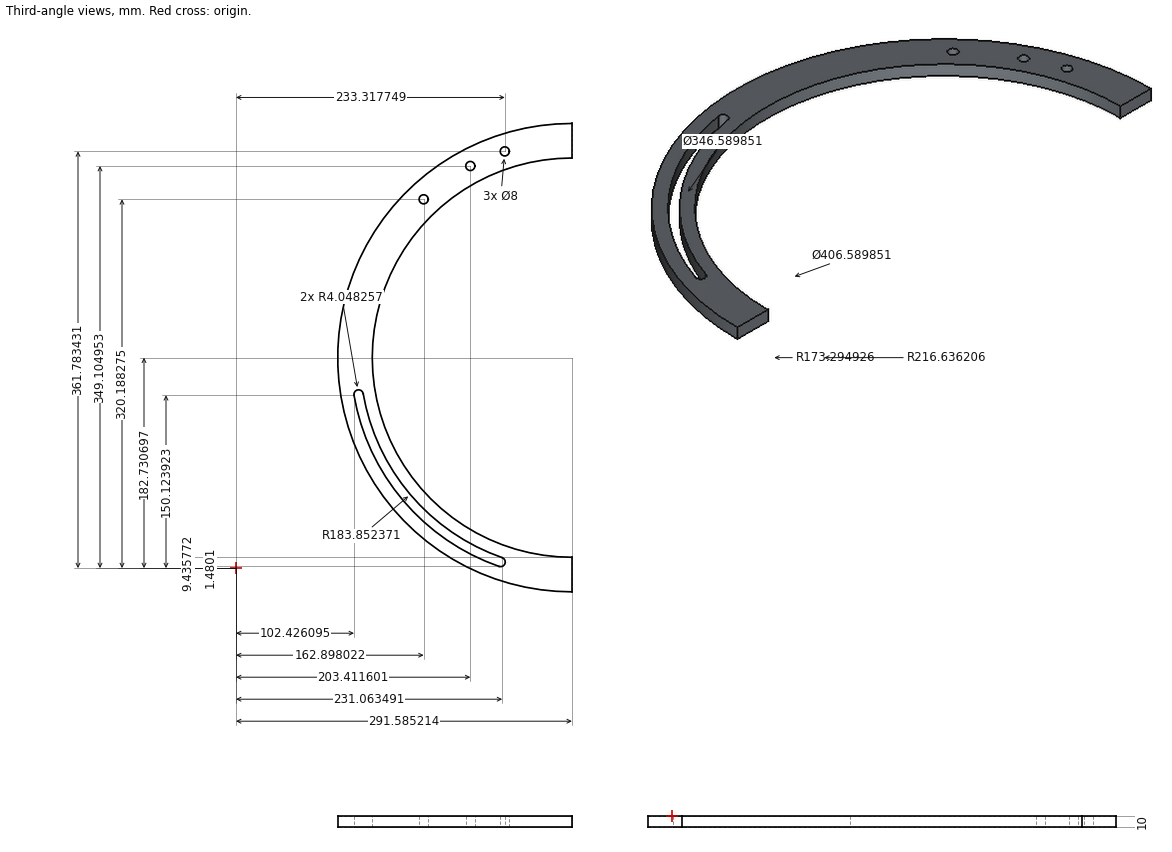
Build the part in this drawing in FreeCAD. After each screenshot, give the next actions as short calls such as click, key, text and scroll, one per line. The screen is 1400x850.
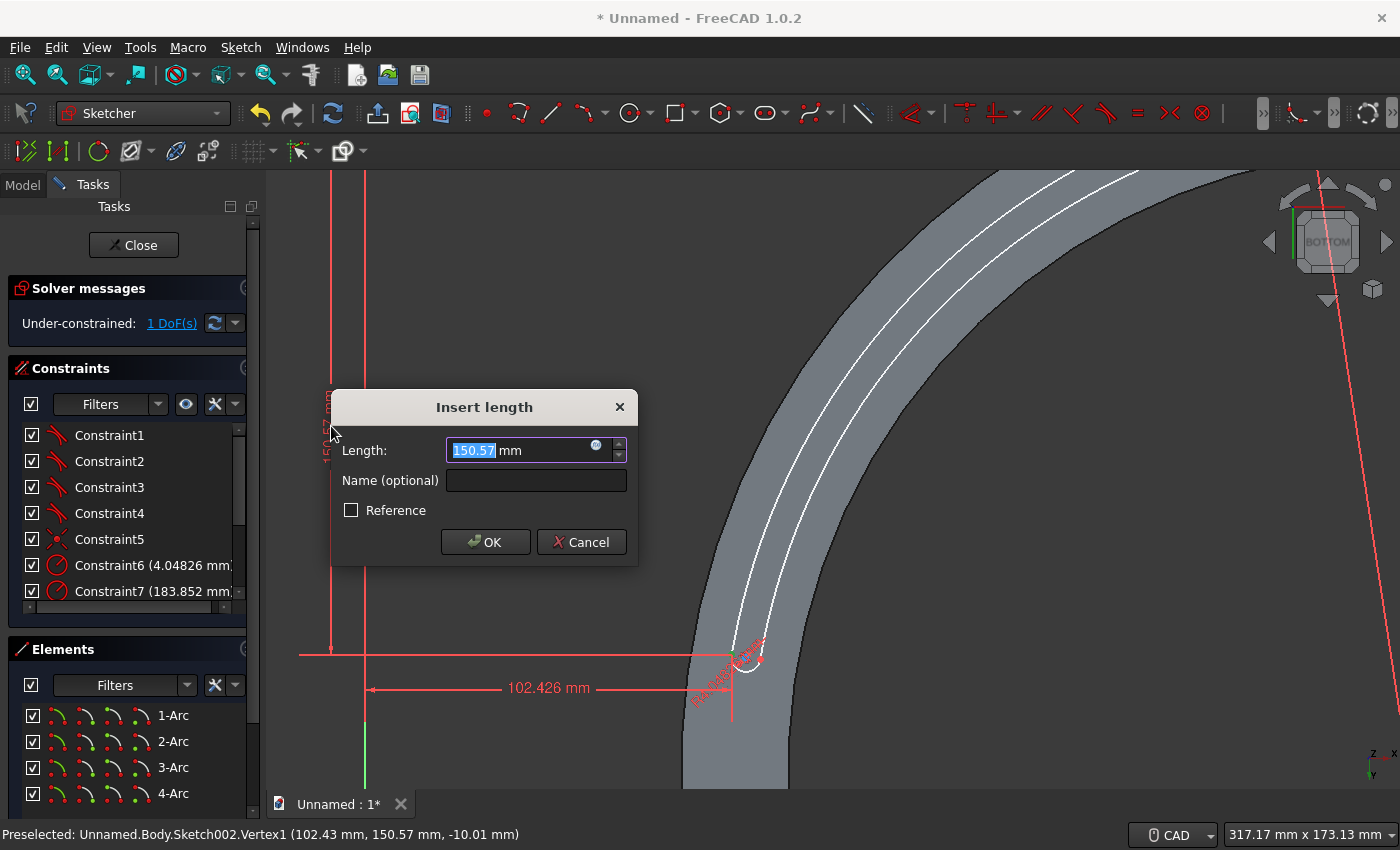
text(150.123923)
key(Return)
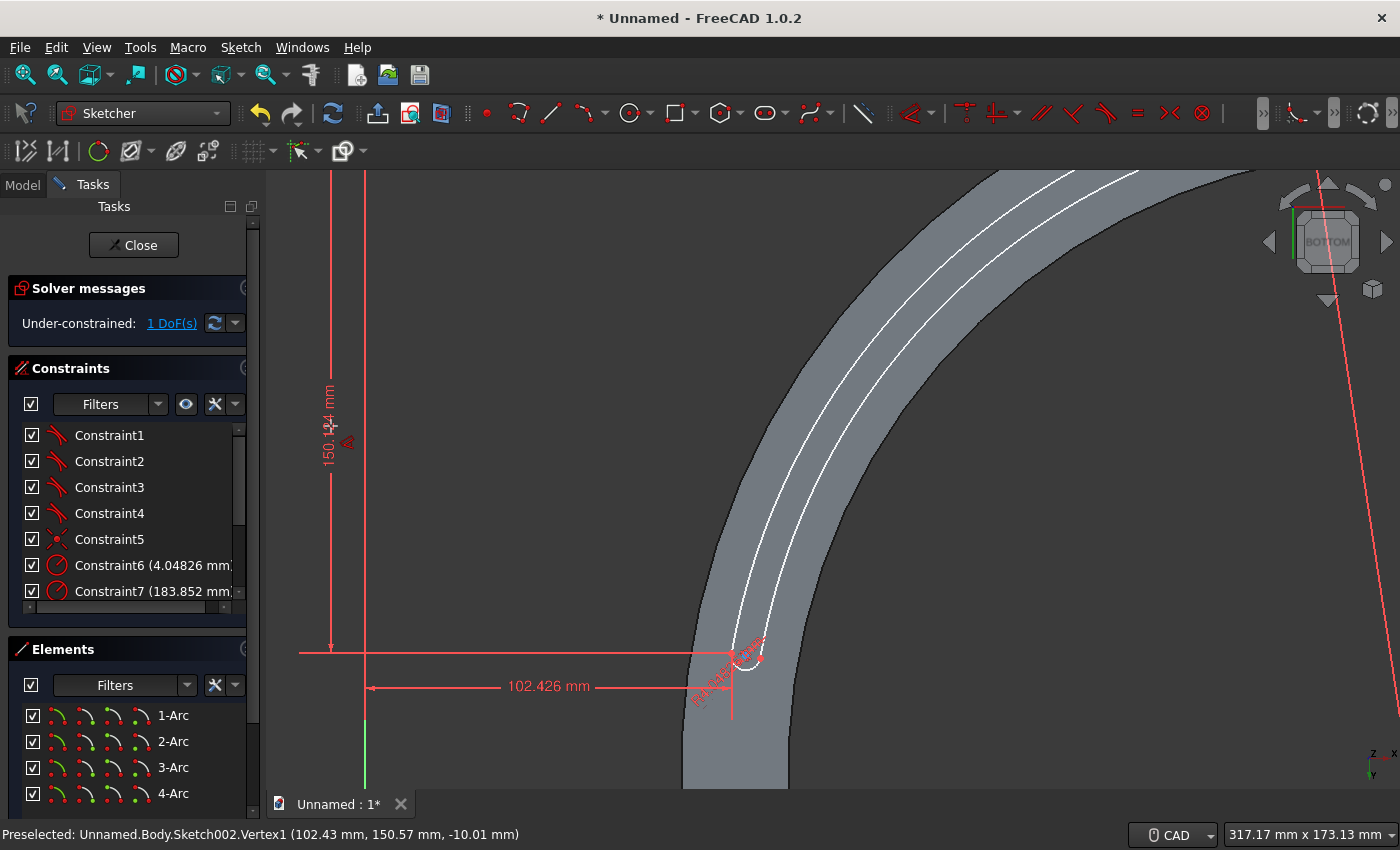
scroll(727, 655, down, 2)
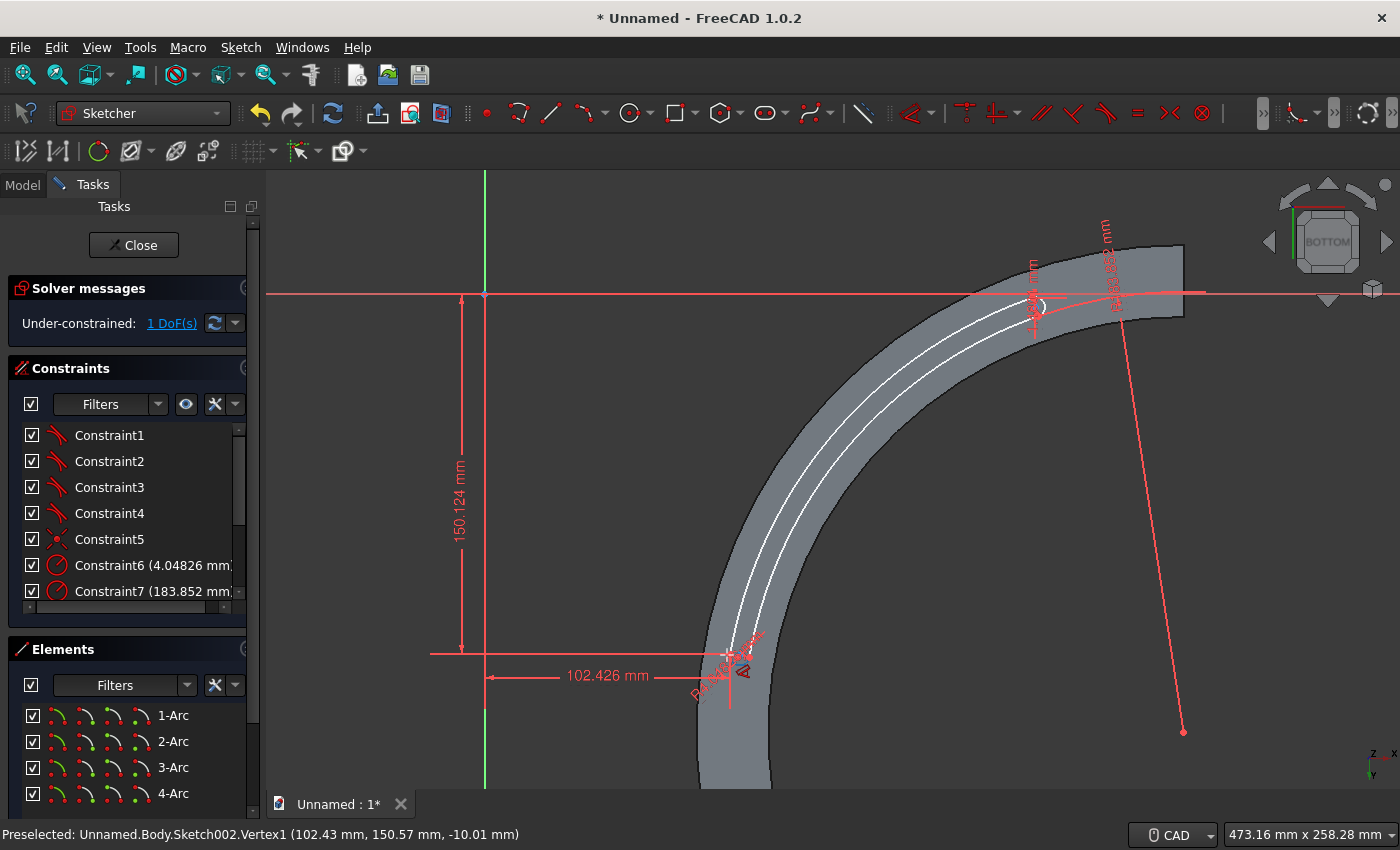
scroll(1039, 316, up, 2)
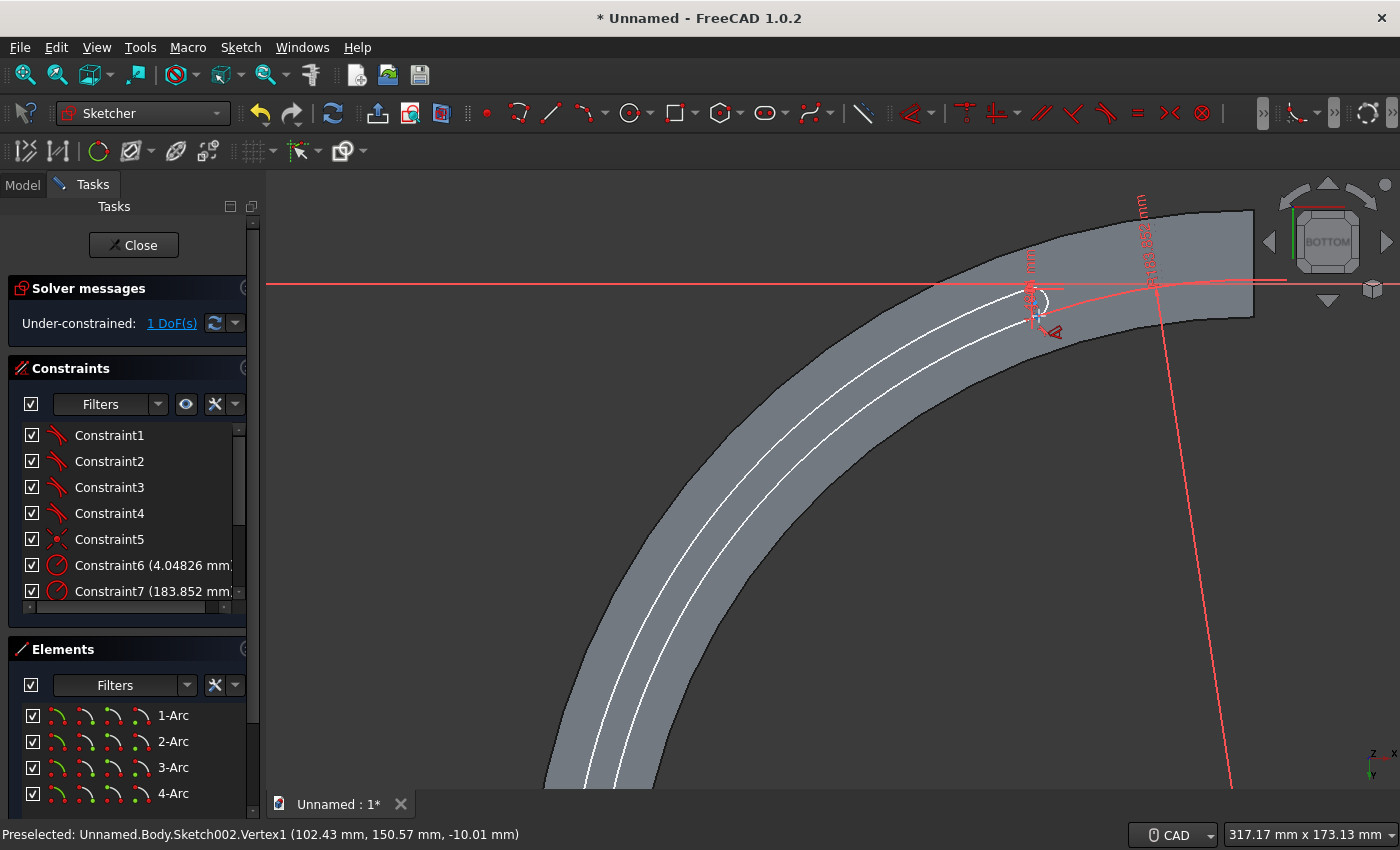
click(1038, 316)
click(666, 250)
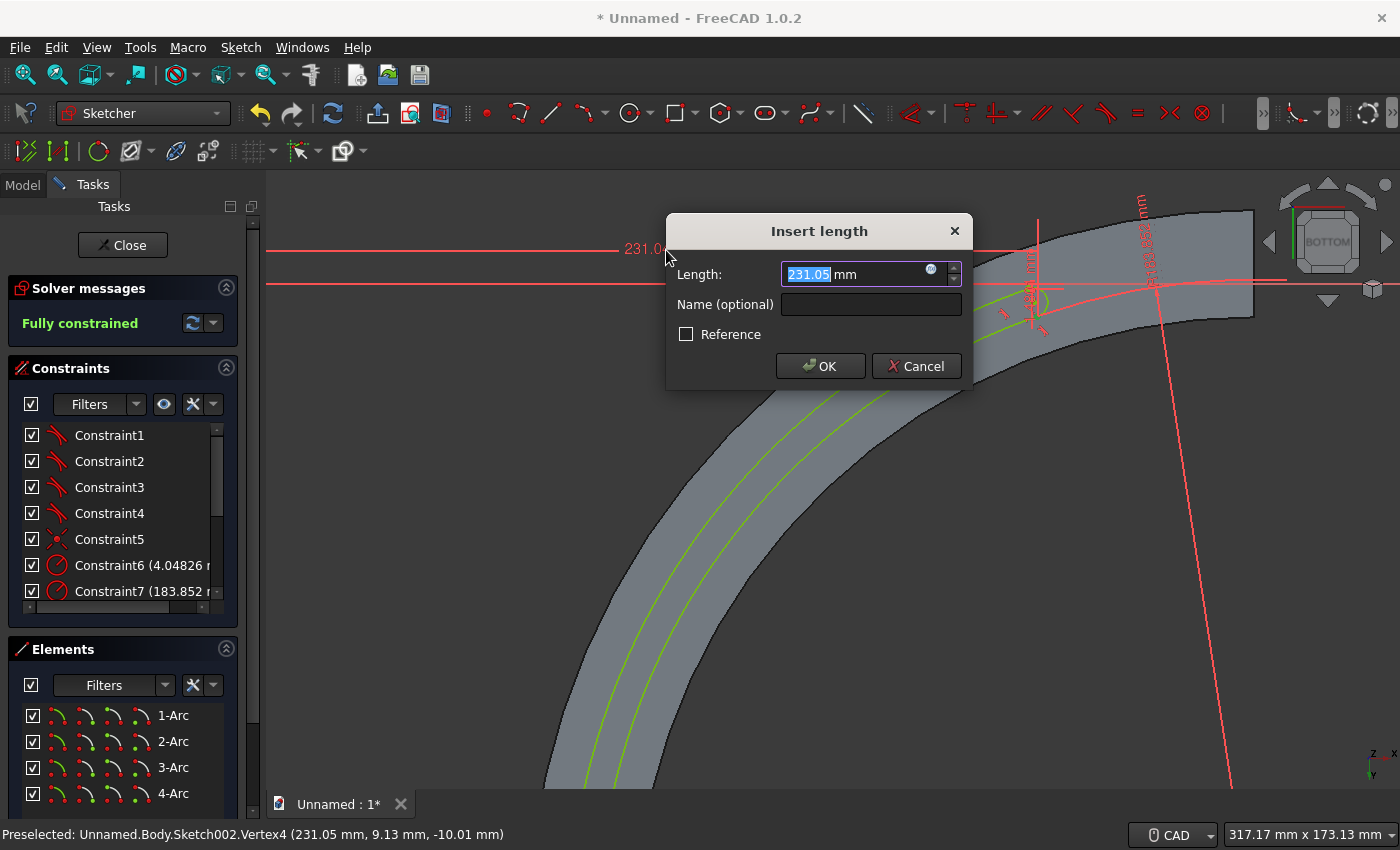
text(231.063491)
key(Return)
key(Escape)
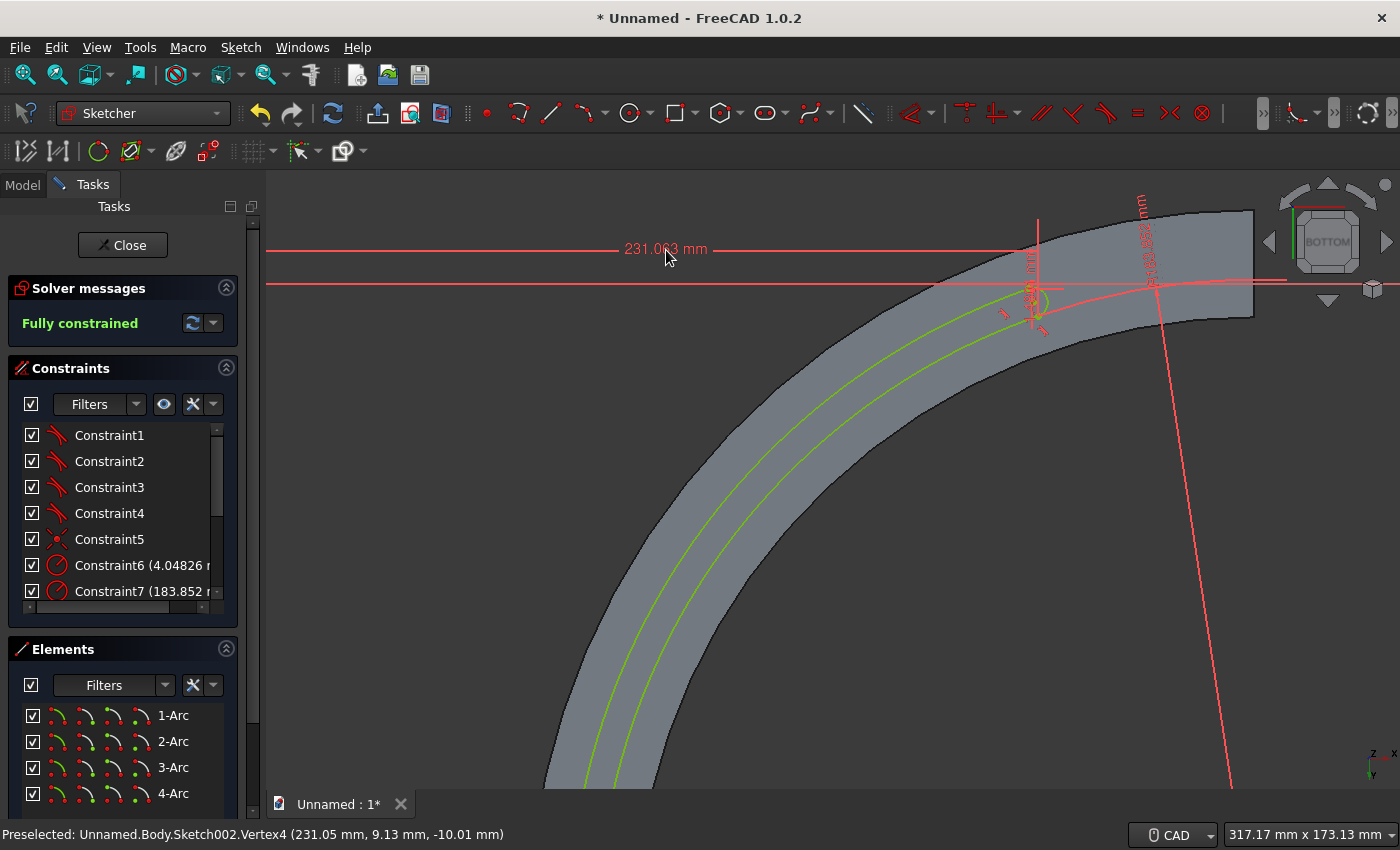
click(123, 245)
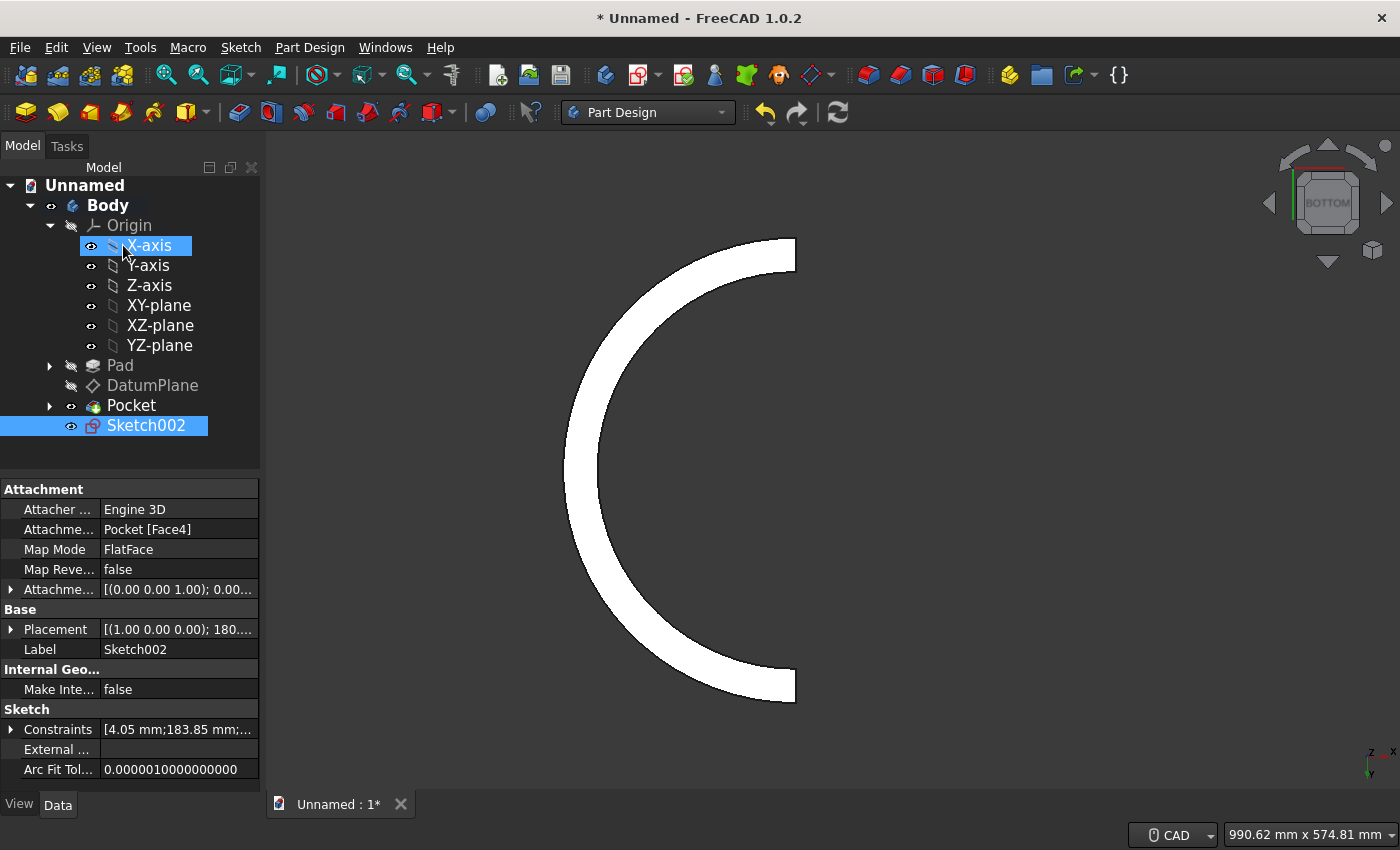
click(240, 112)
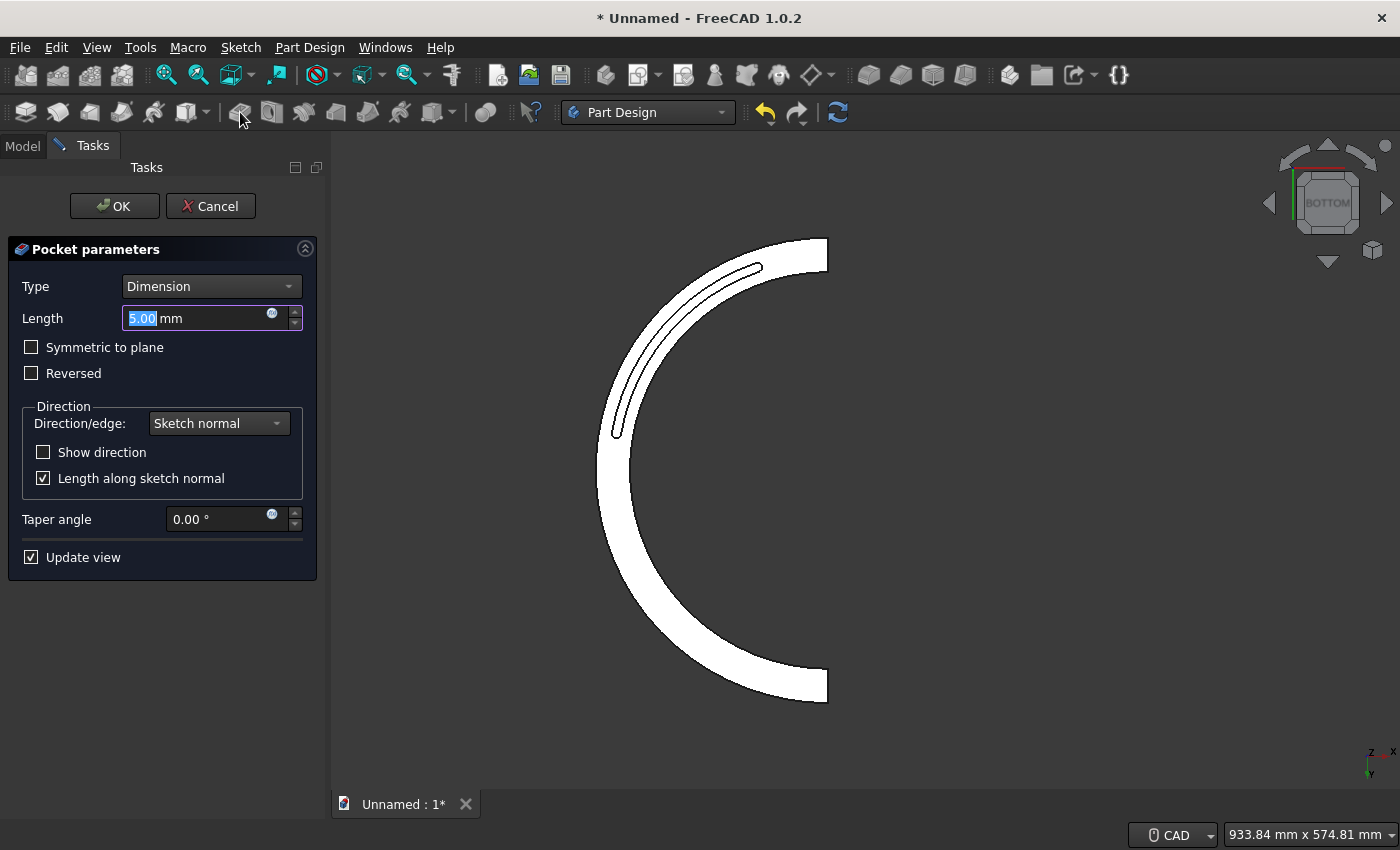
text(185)
key(Tab)